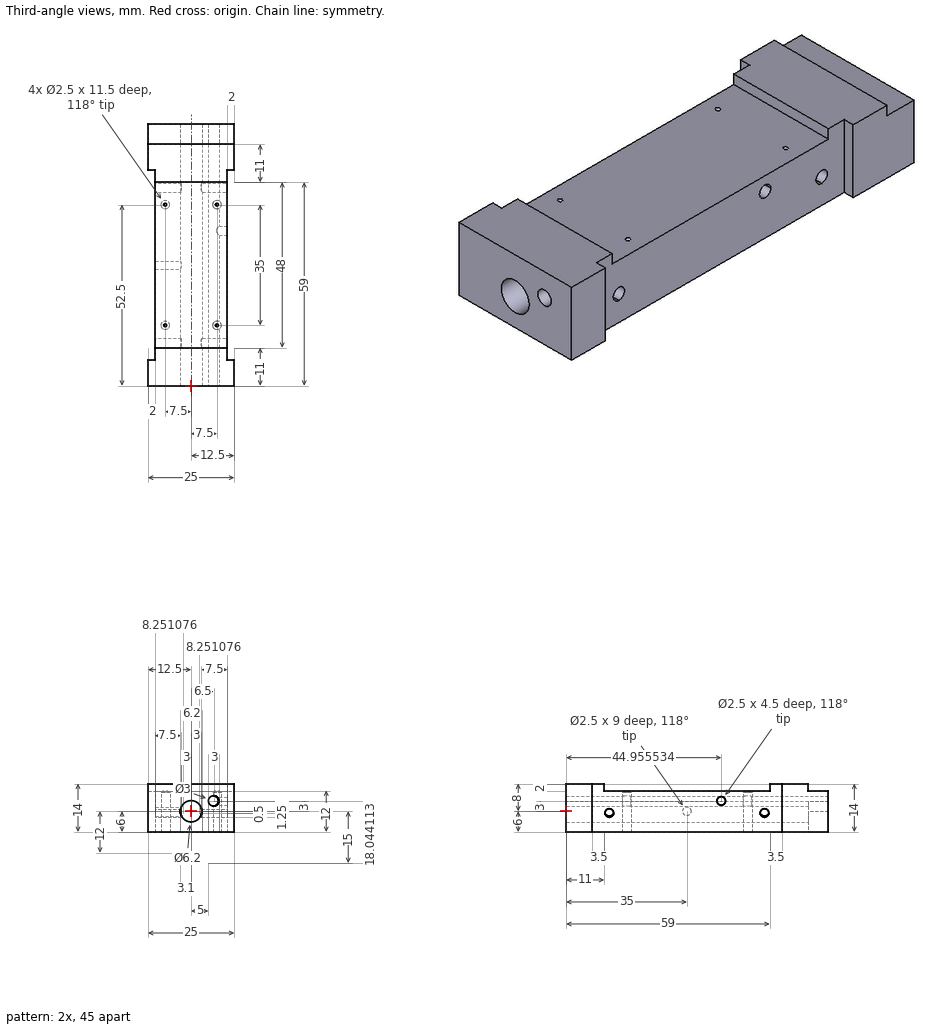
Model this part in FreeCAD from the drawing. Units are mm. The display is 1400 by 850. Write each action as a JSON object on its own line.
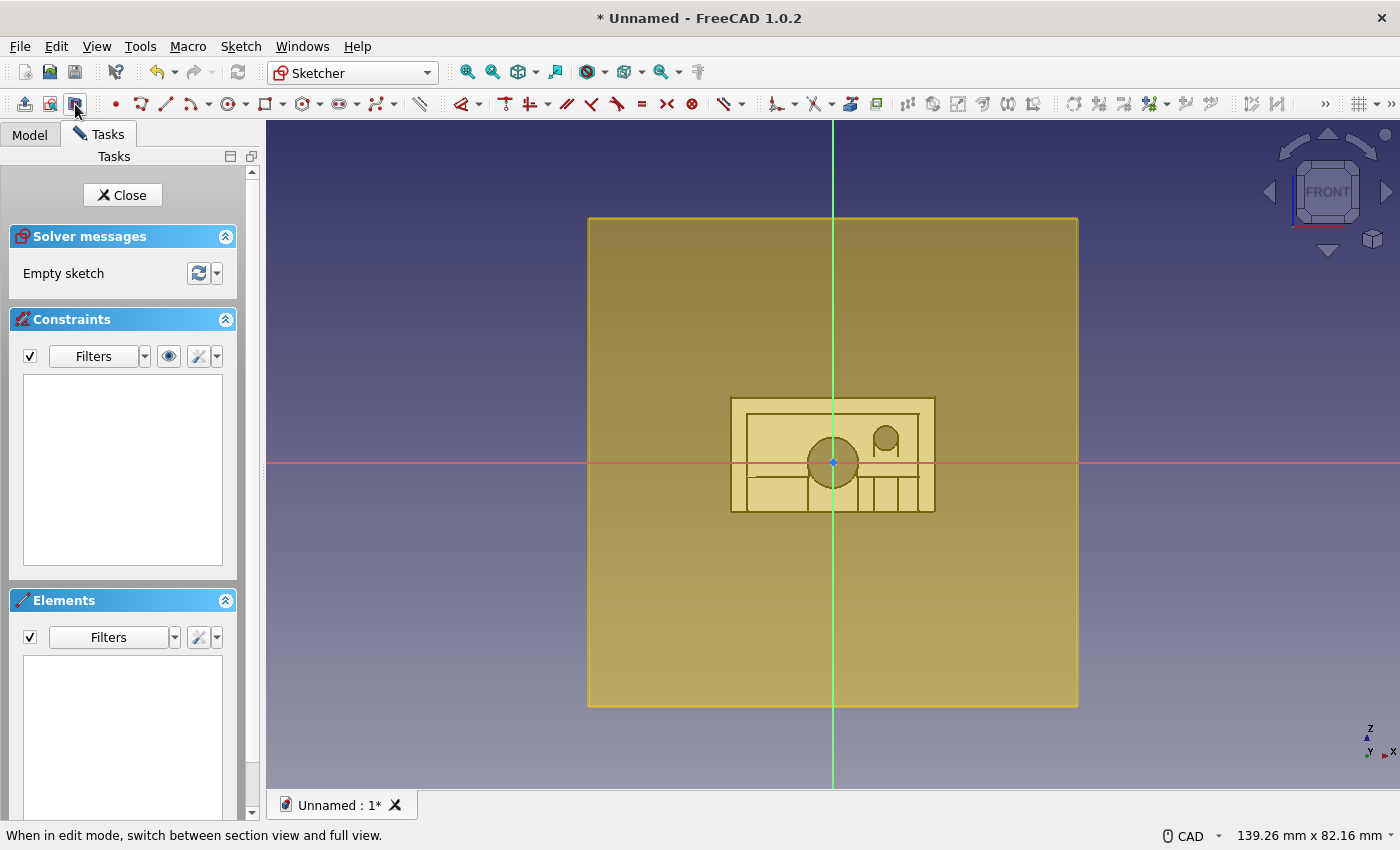
{"action": "scroll", "coordinate": [779, 473], "scroll_direction": "up", "scroll_amount": 9}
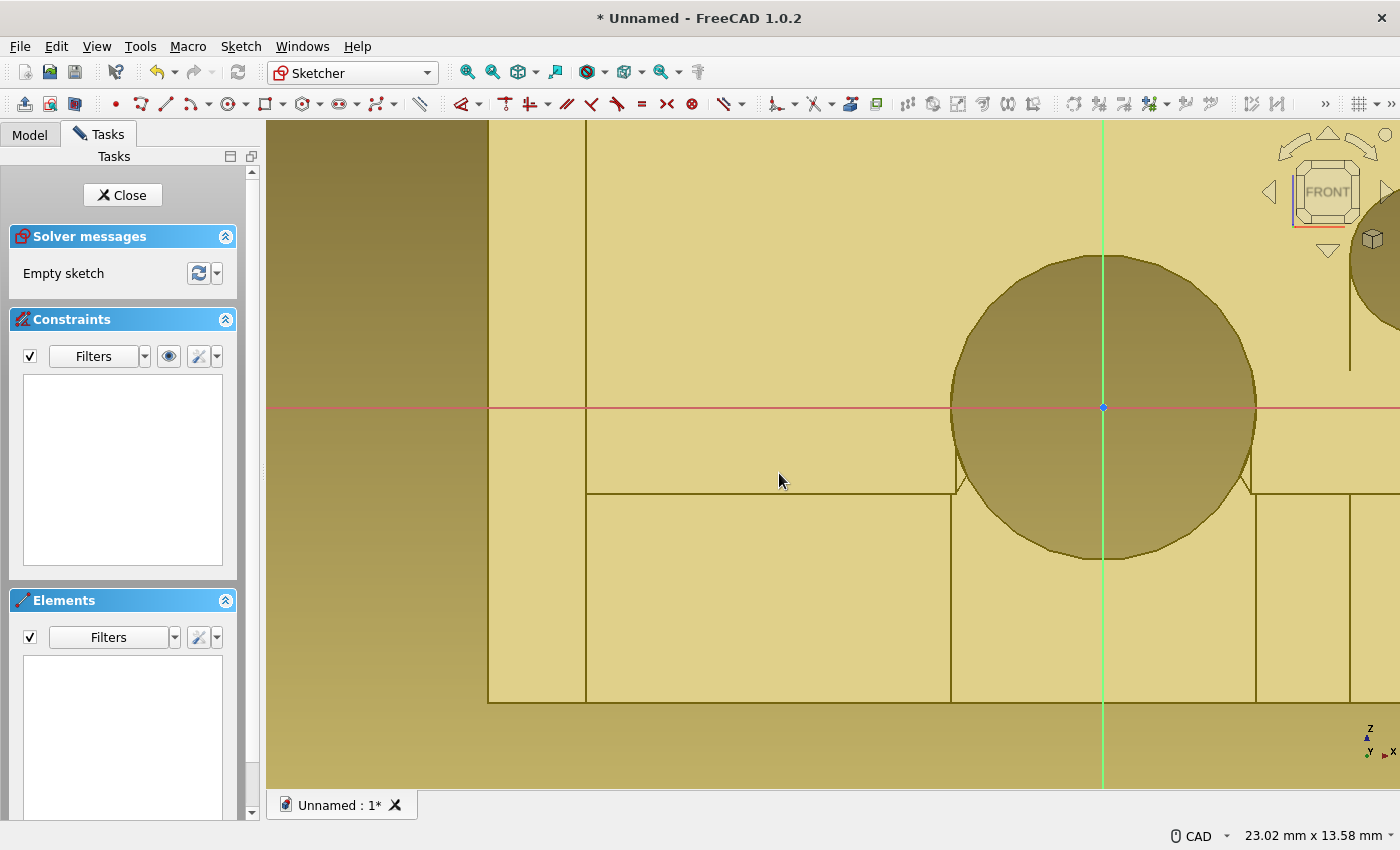
{"action": "left_click", "coordinate": [141, 104]}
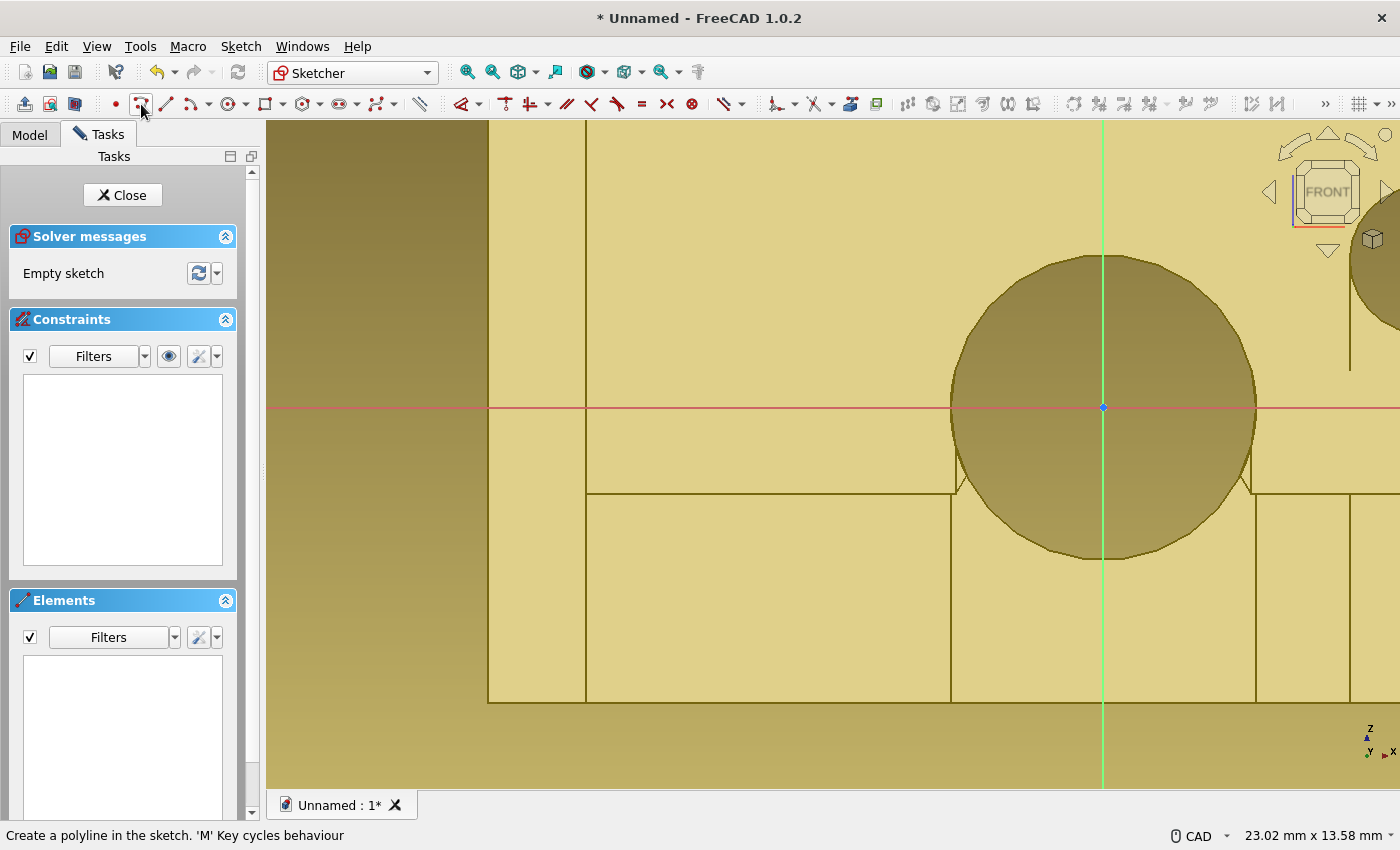
{"action": "left_click", "coordinate": [993, 432]}
{"action": "left_click", "coordinate": [956, 494]}
{"action": "left_click", "coordinate": [586, 494]}
{"action": "left_click", "coordinate": [586, 432]}
{"action": "left_click", "coordinate": [993, 433]}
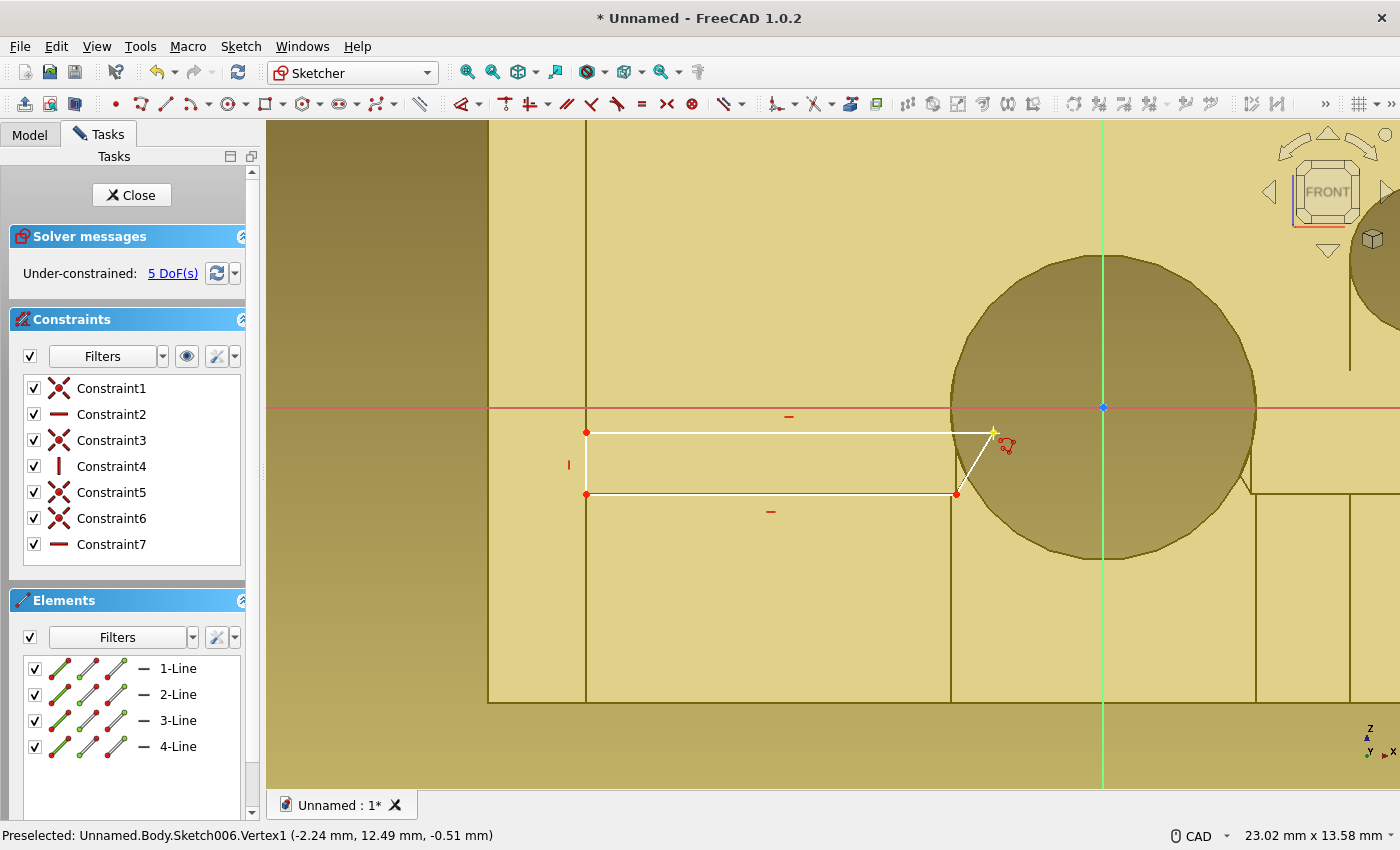
{"action": "left_click", "coordinate": [166, 104]}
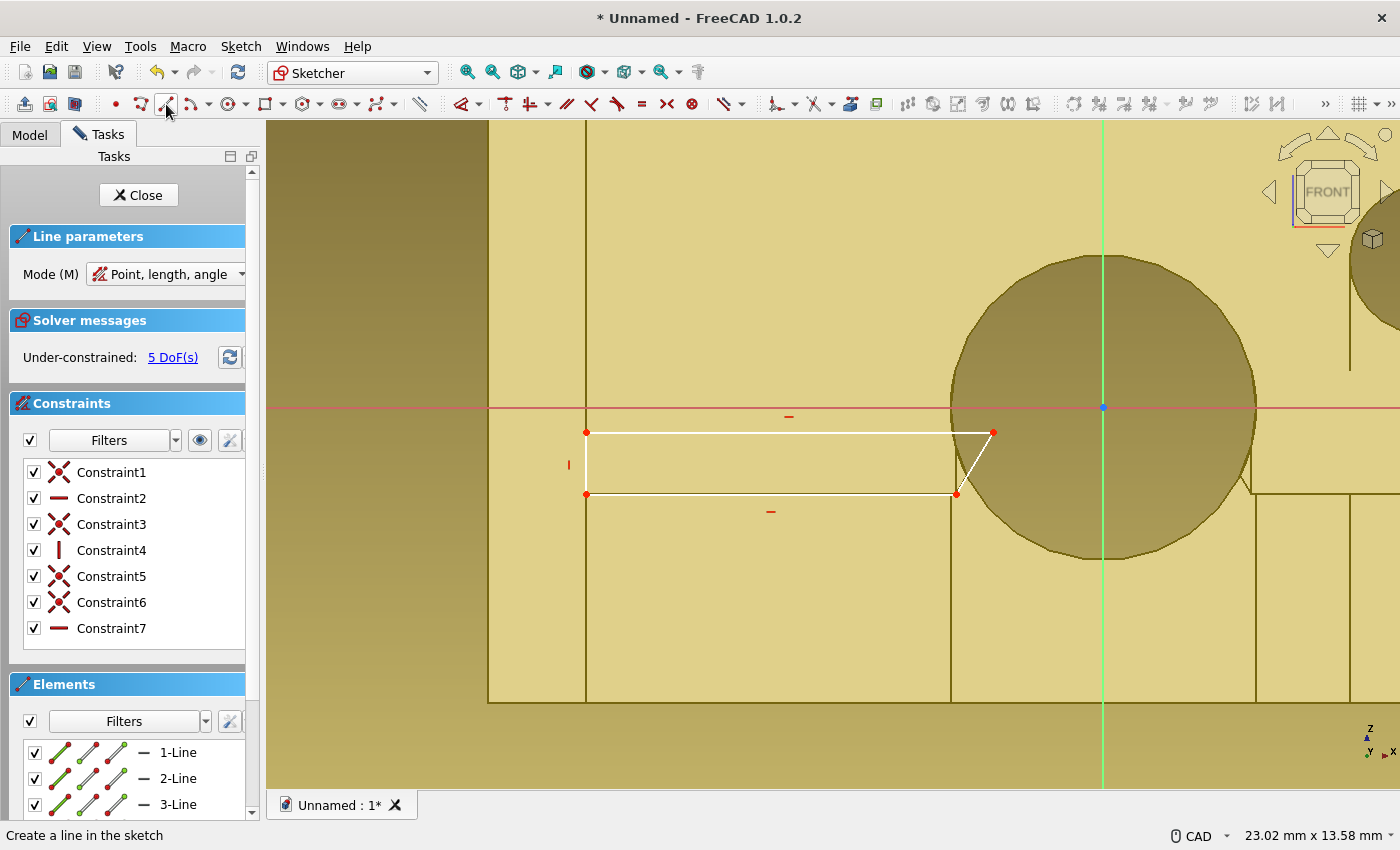
{"action": "left_click", "coordinate": [546, 432]}
{"action": "left_click", "coordinate": [424, 432]}
{"action": "key", "text": "Escape"}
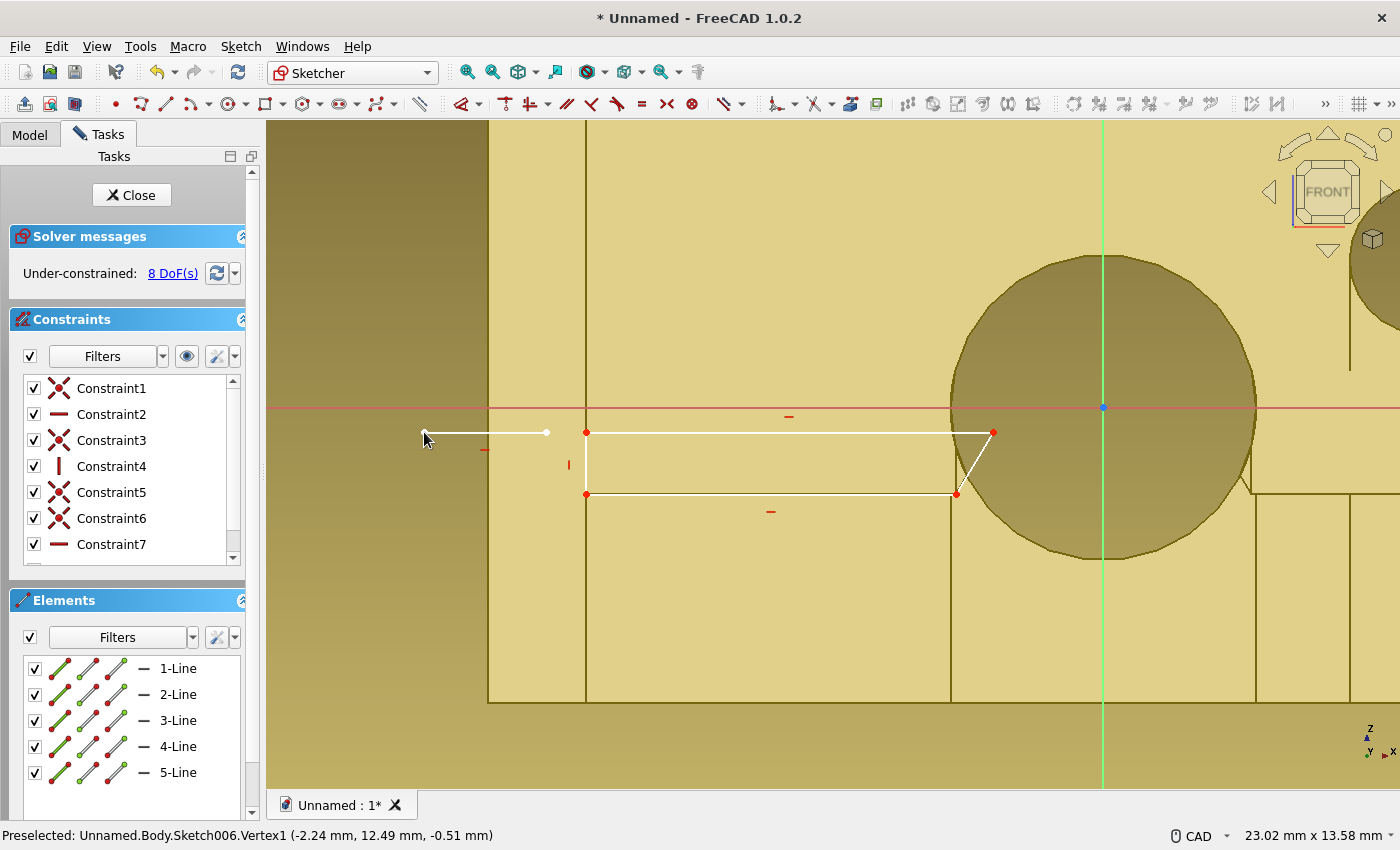
{"action": "left_click", "coordinate": [509, 433]}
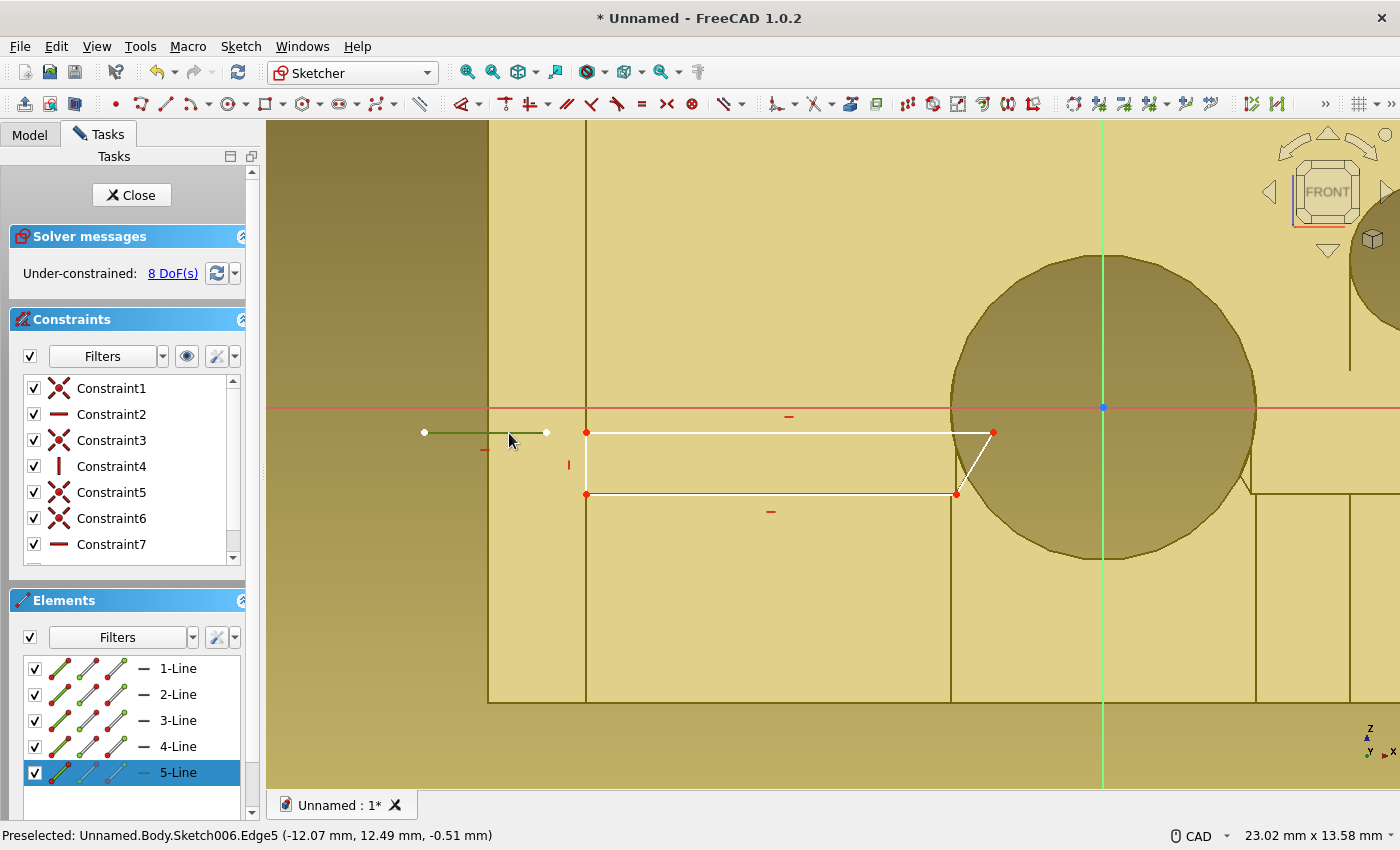
{"action": "left_click", "coordinate": [420, 104]}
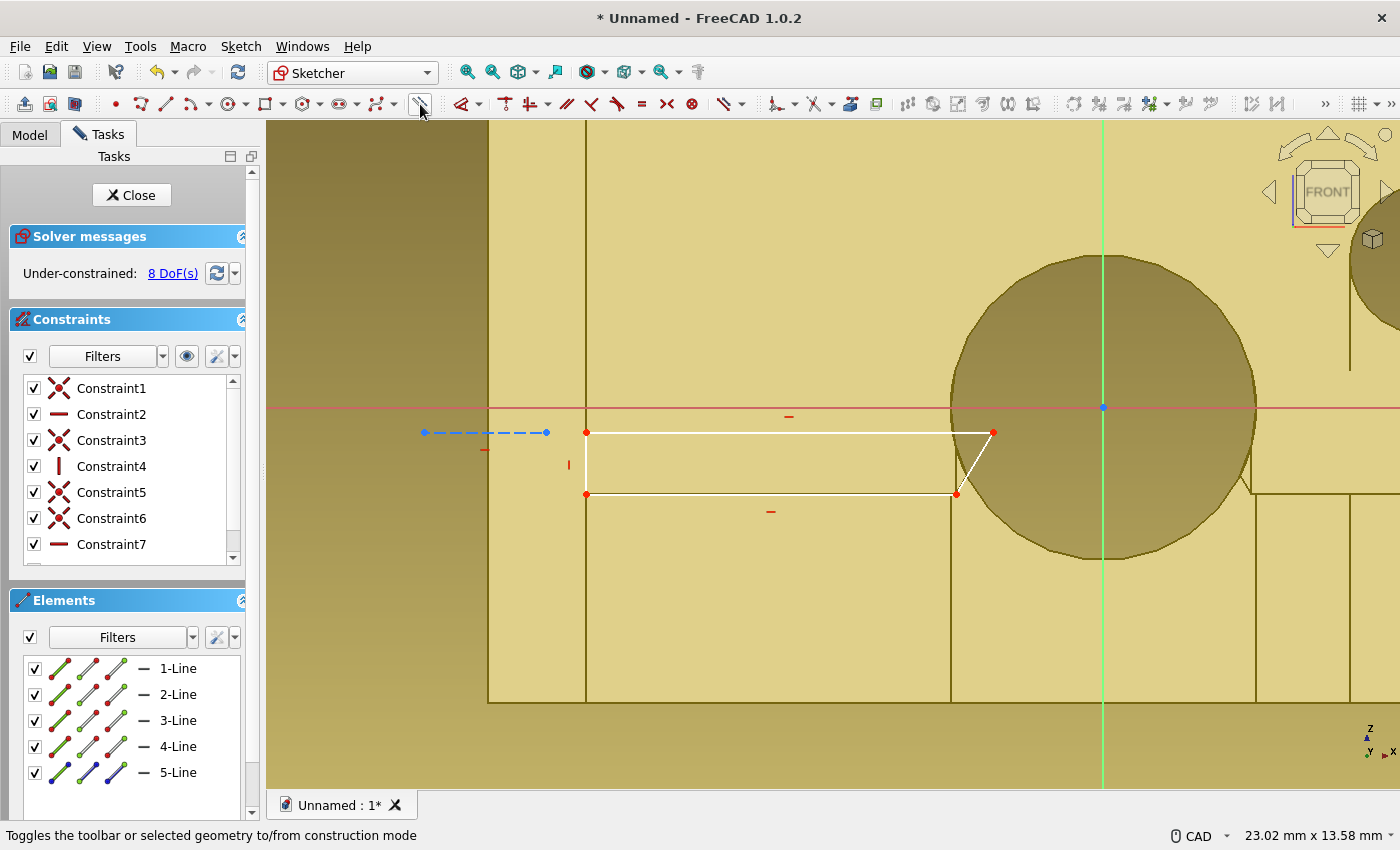
{"action": "left_click", "coordinate": [460, 104]}